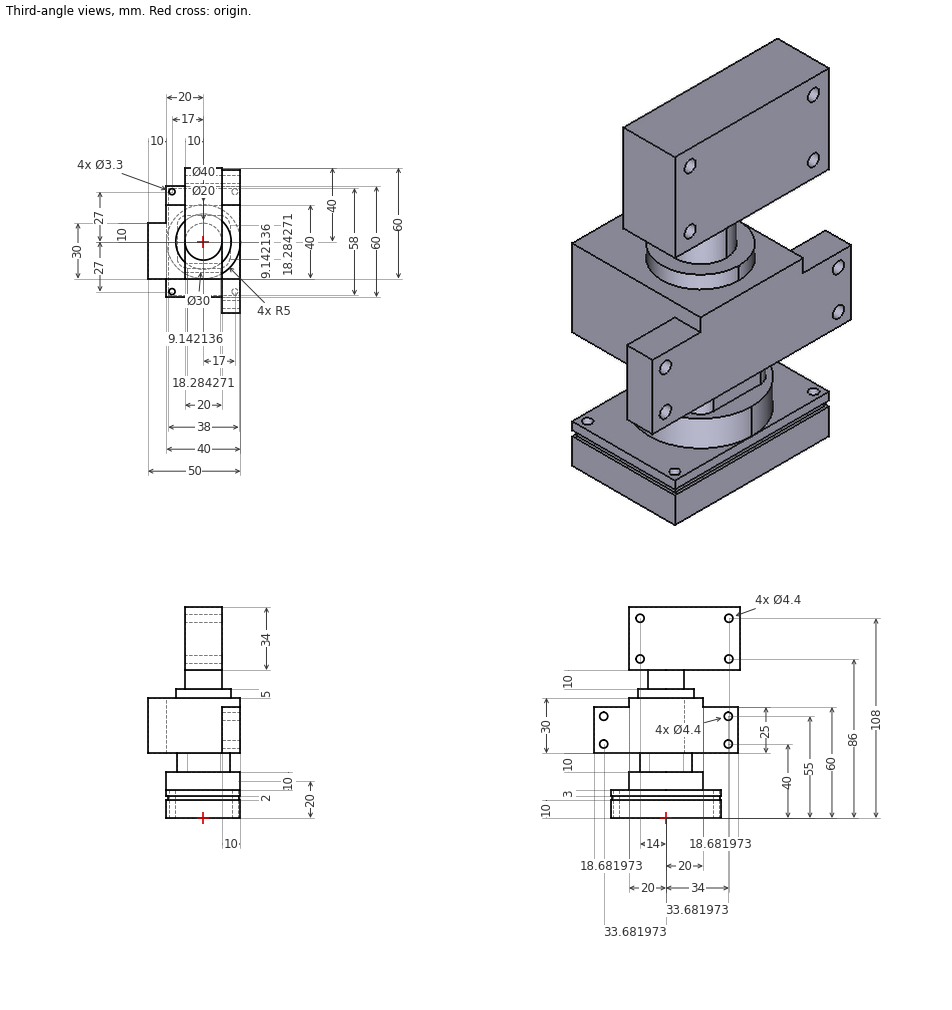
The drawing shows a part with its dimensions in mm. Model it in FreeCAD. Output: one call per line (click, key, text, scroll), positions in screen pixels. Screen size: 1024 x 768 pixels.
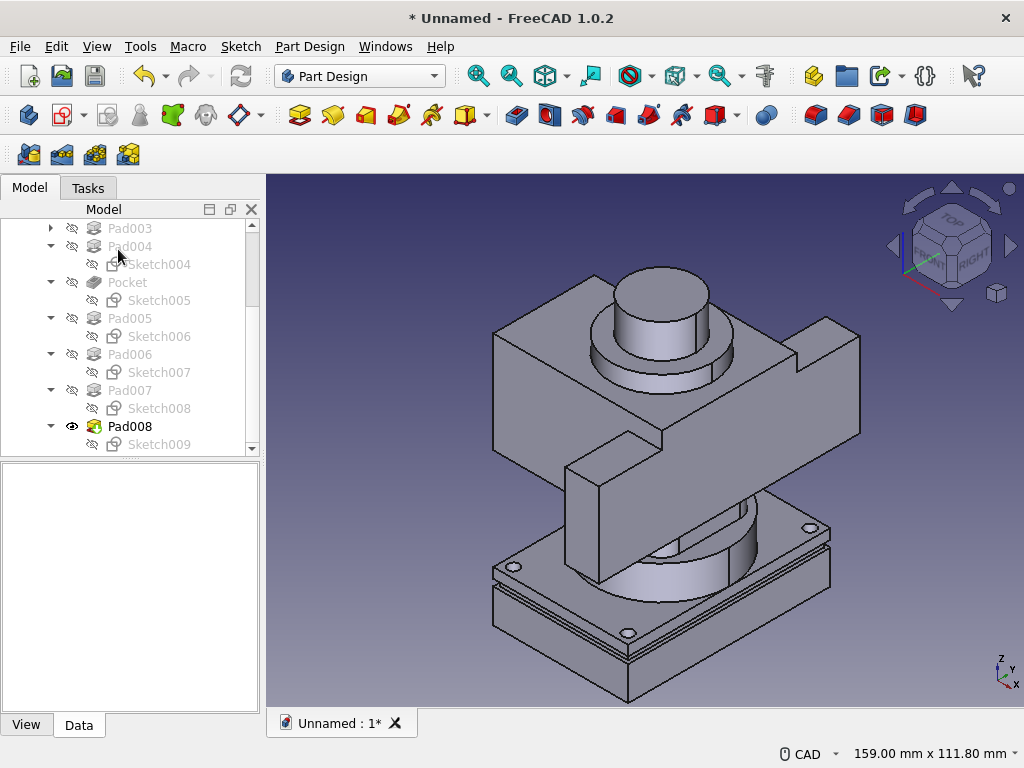
key(v)
key(f)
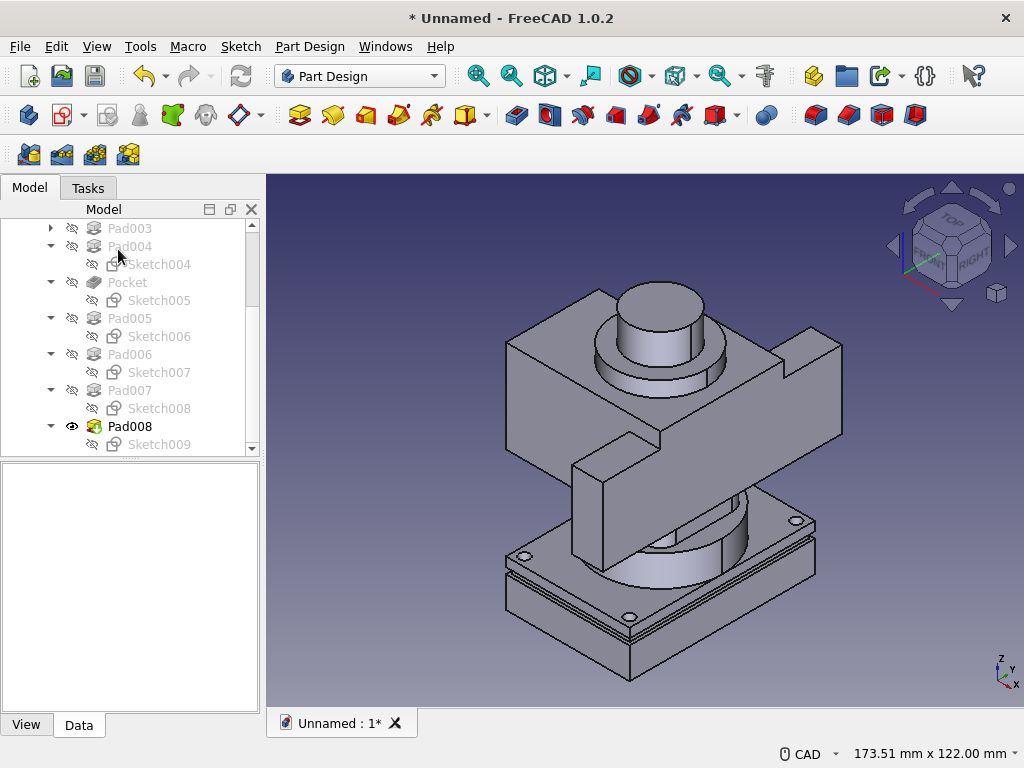
key(6)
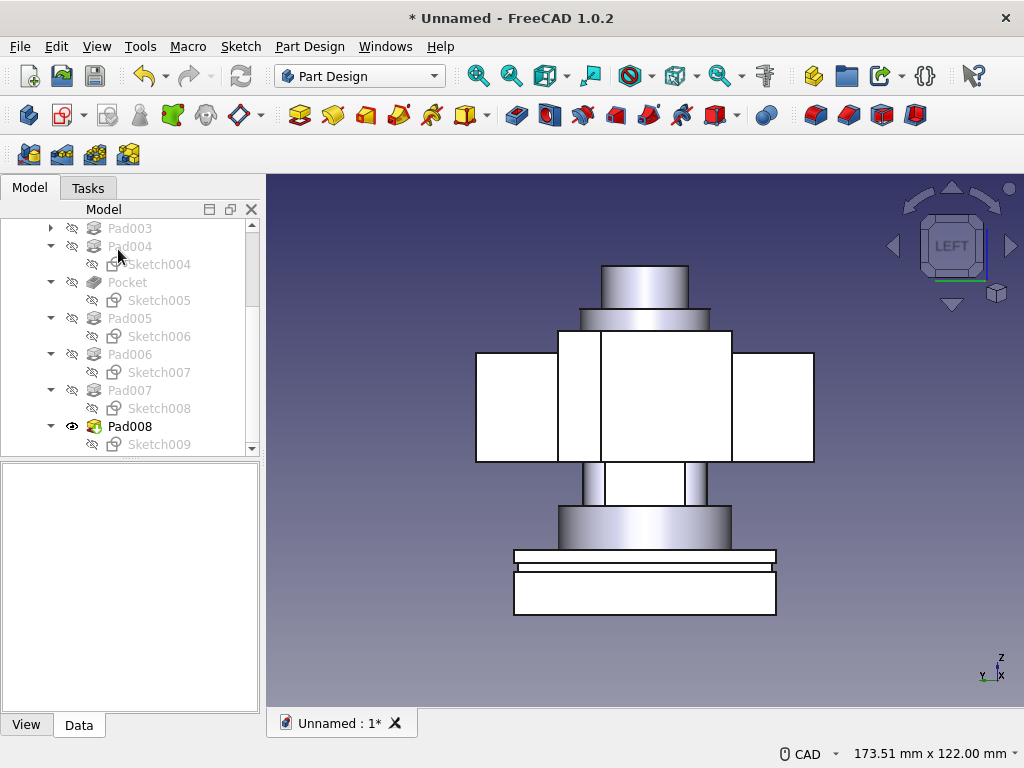
click(517, 407)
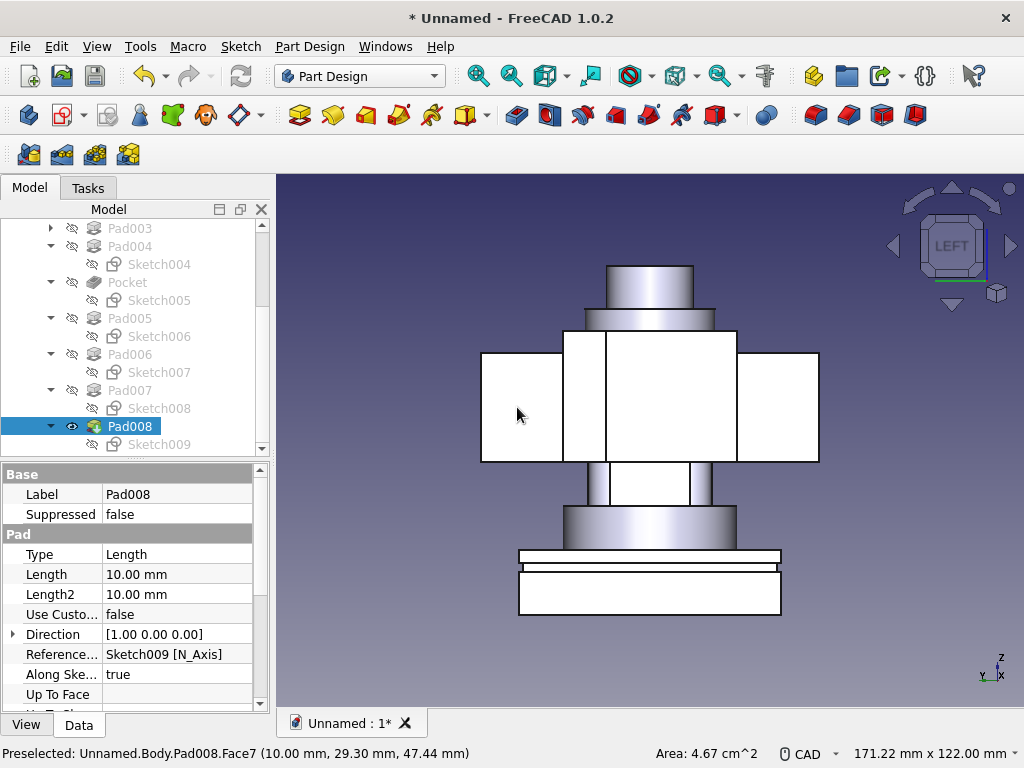
click(62, 116)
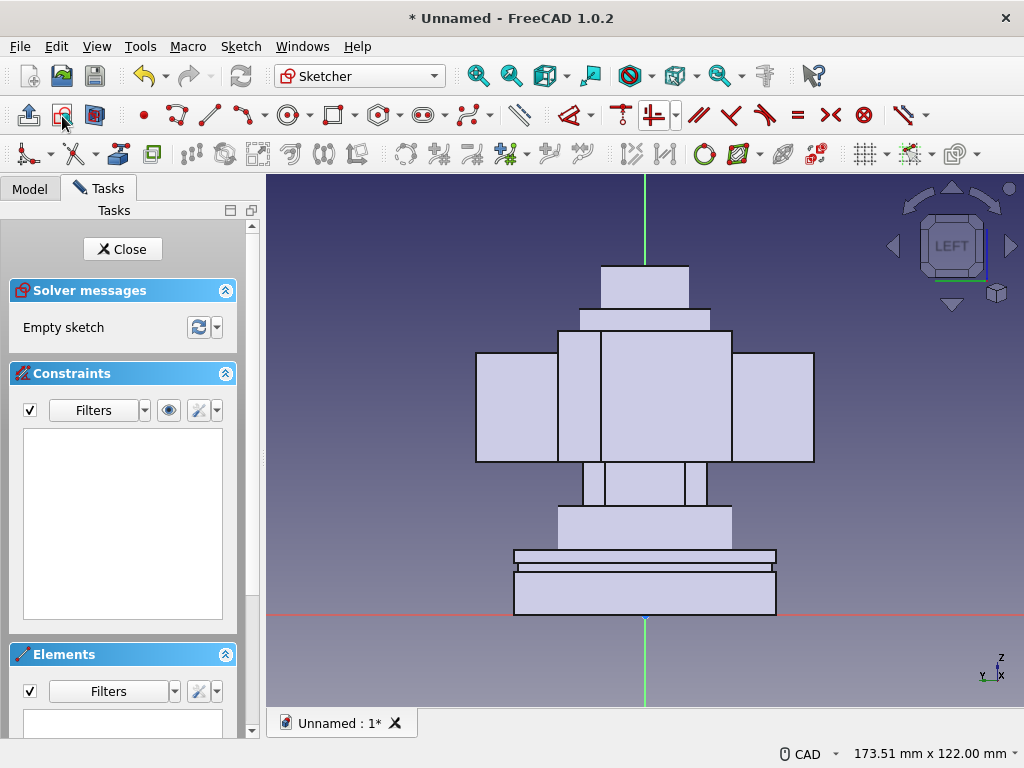
key(q)
key(s)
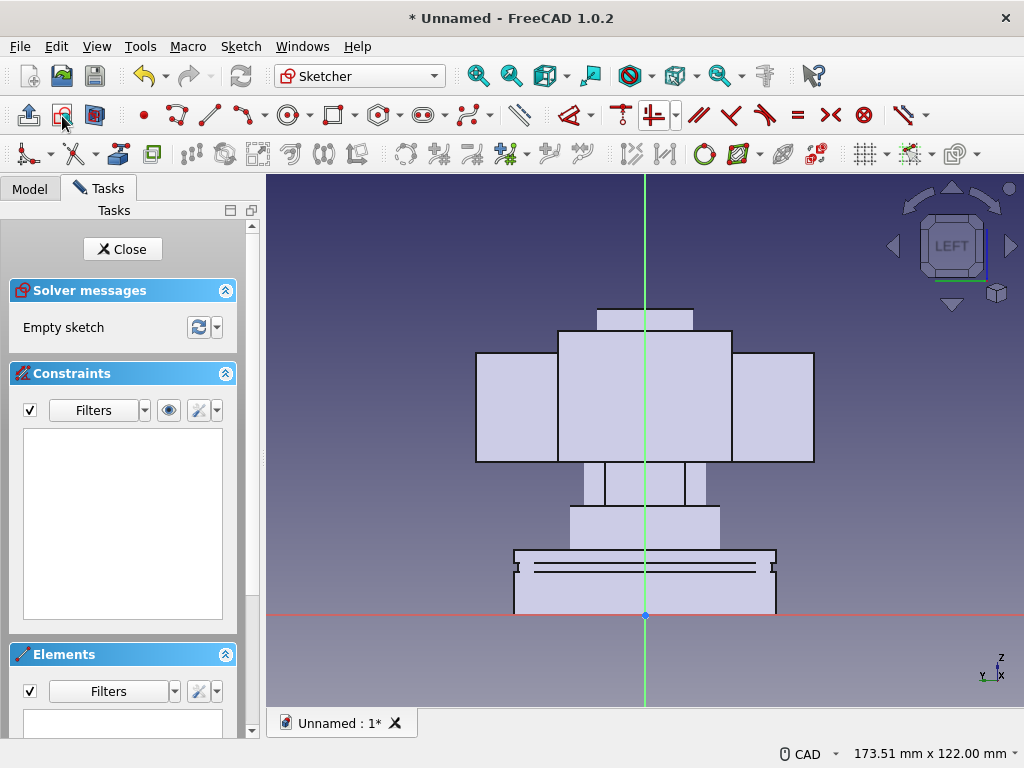
key(g)
key(c)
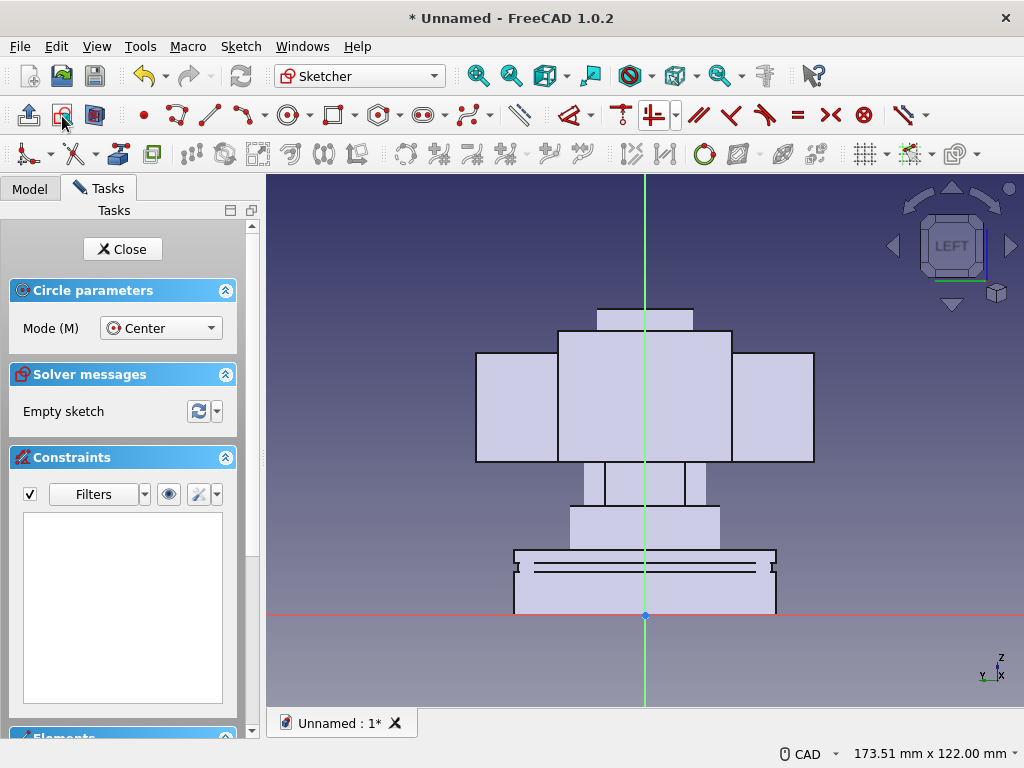
scroll(498, 375, up, 5)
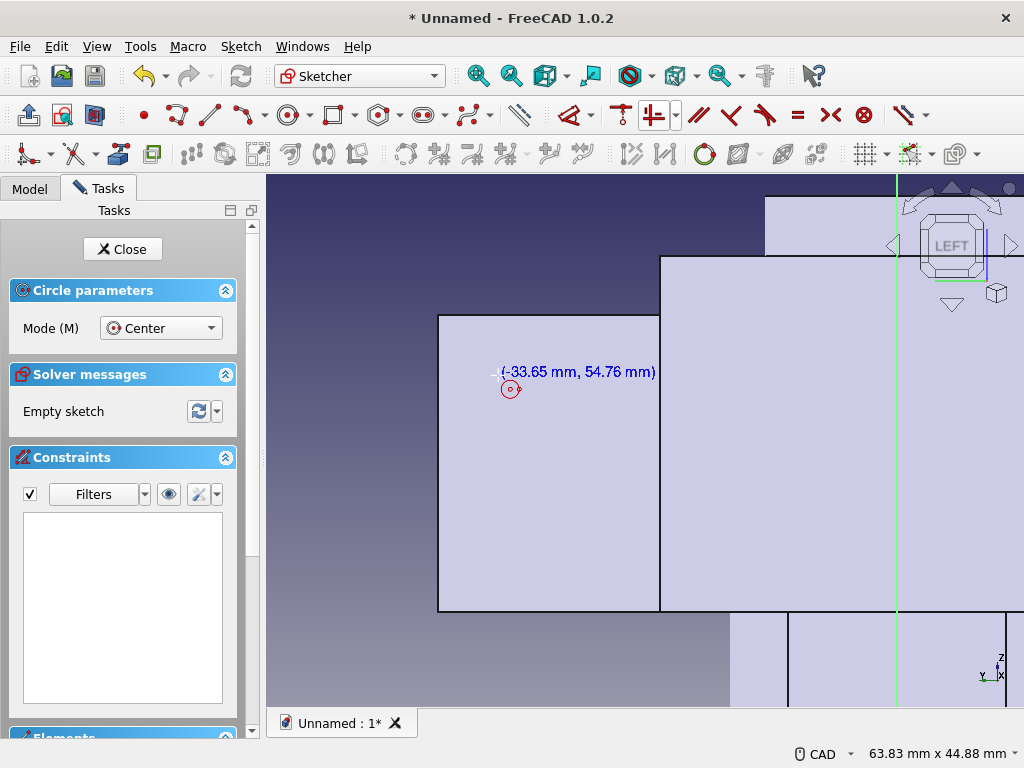
click(497, 374)
move(516, 356)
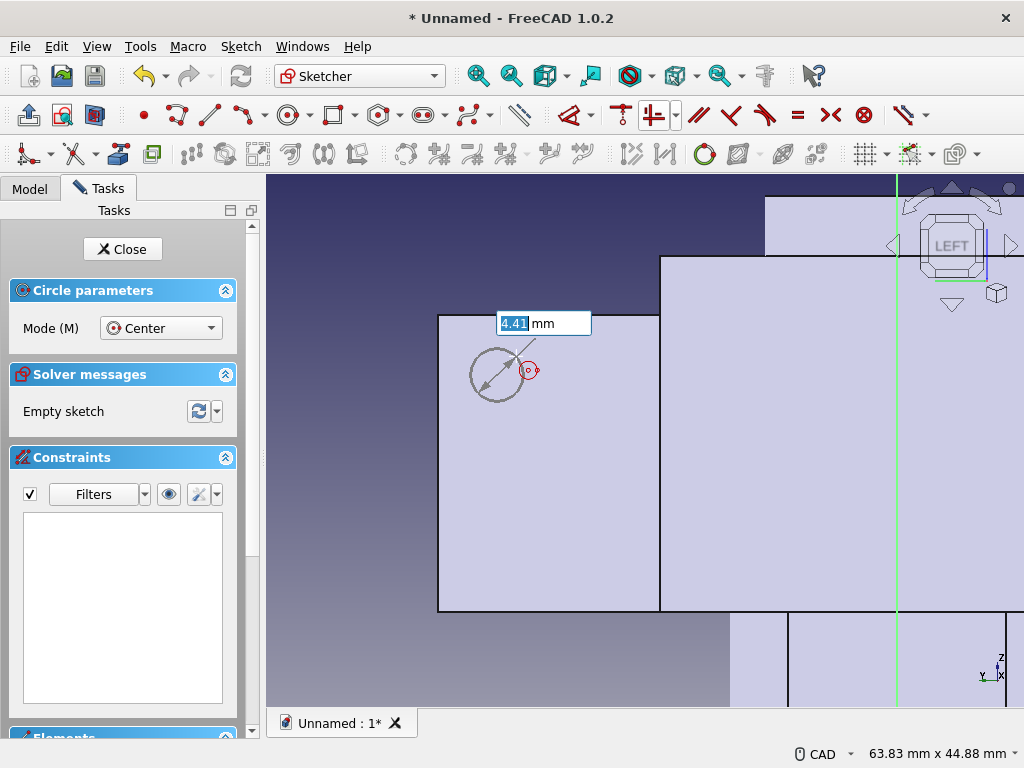
text(4.4)
key(Return)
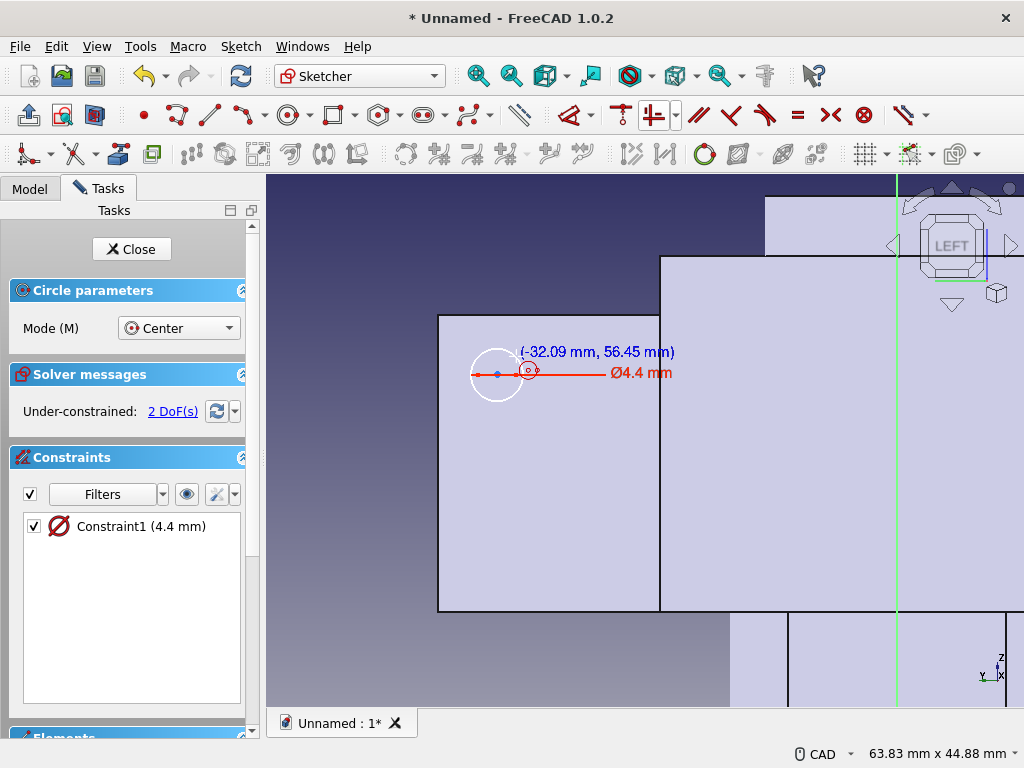
click(497, 552)
move(516, 534)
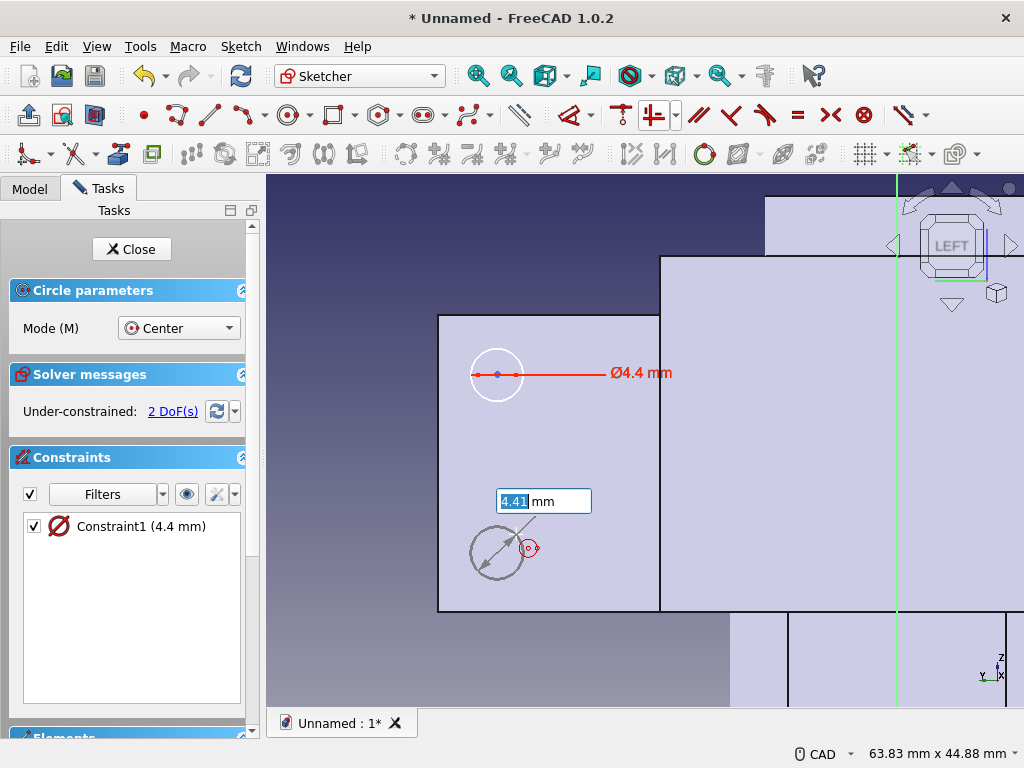
text(4.4)
key(Return)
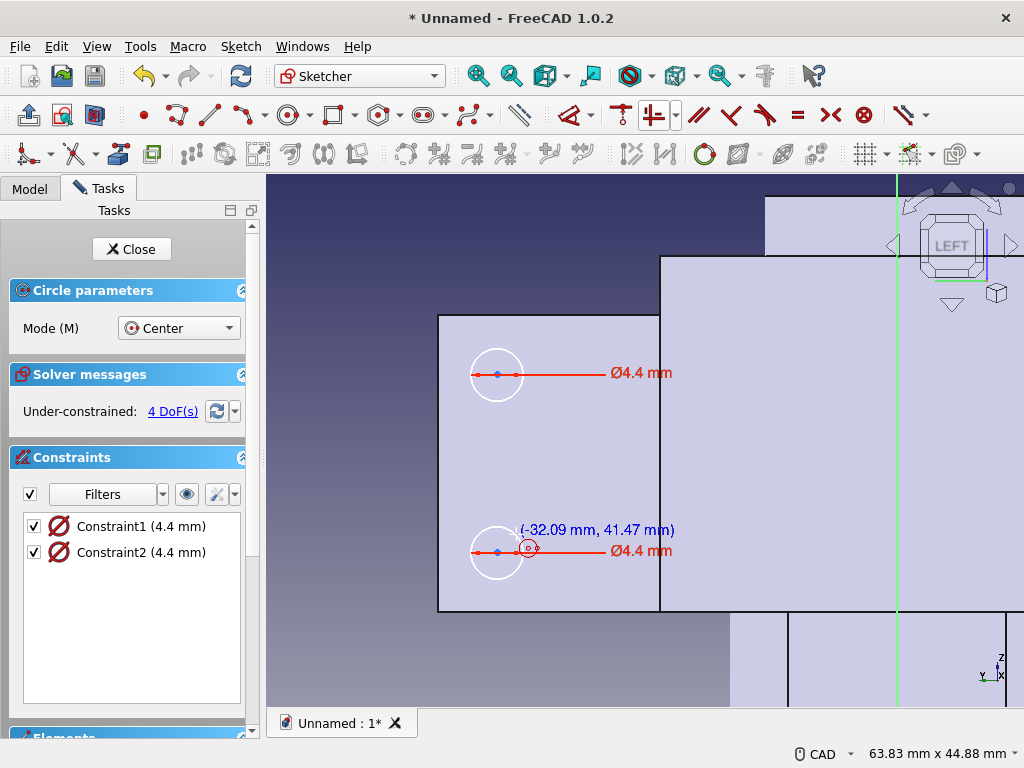
scroll(315, 239, down, 4)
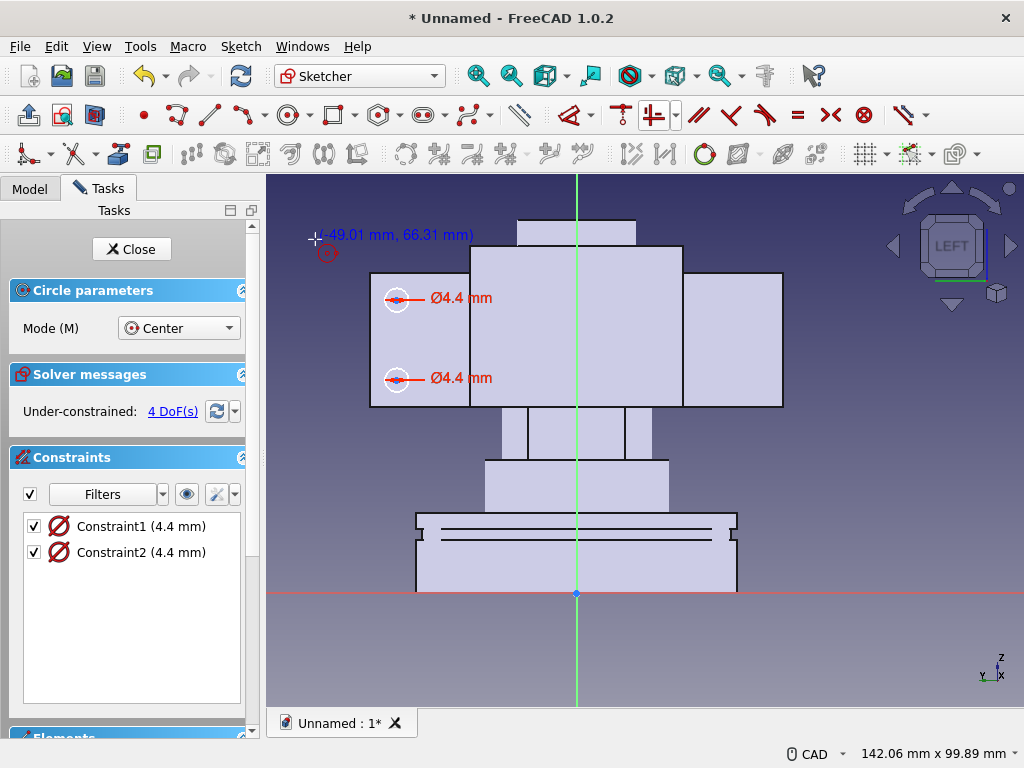
scroll(756, 380, up, 4)